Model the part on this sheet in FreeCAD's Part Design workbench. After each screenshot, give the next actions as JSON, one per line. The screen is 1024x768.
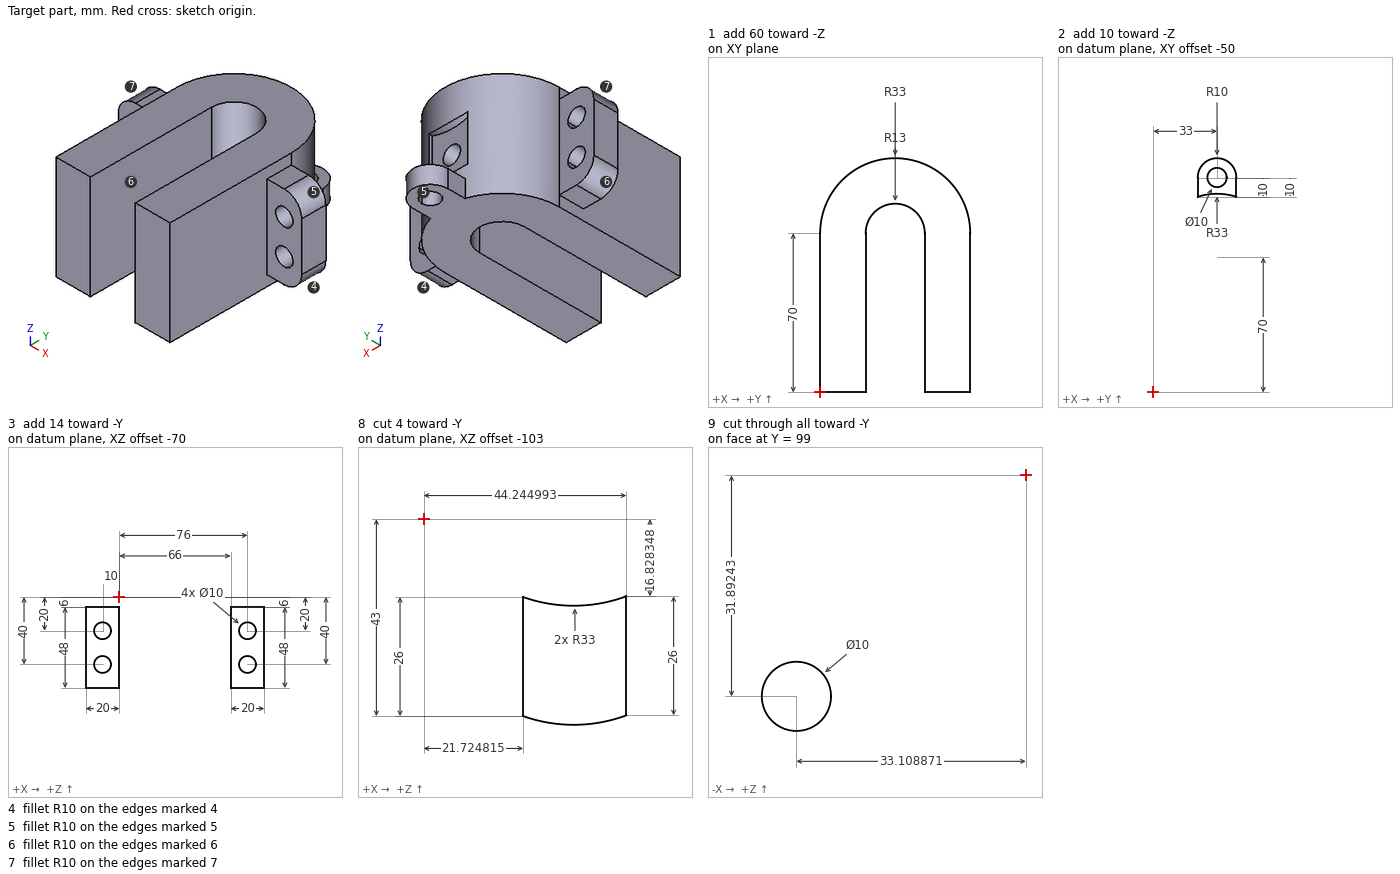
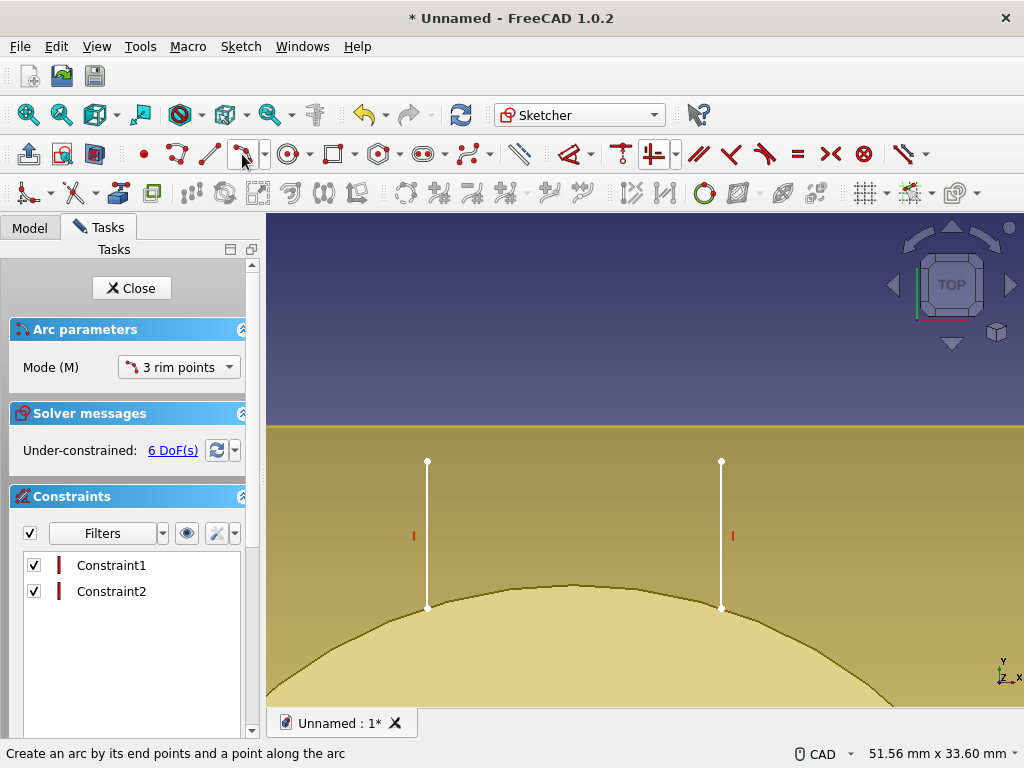
{"action": "left_click", "coordinate": [721, 609]}
{"action": "left_click", "coordinate": [427, 609]}
{"action": "left_click", "coordinate": [574, 585]}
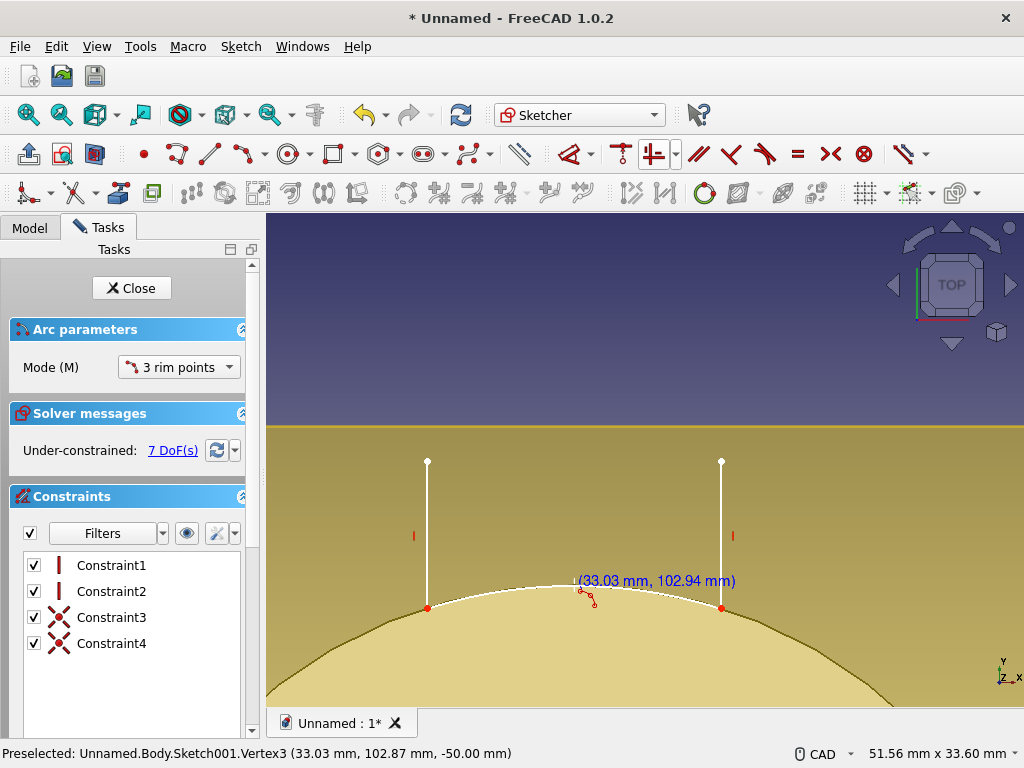
{"action": "left_click", "coordinate": [427, 462]}
{"action": "left_click", "coordinate": [721, 462]}
{"action": "left_click", "coordinate": [574, 314]}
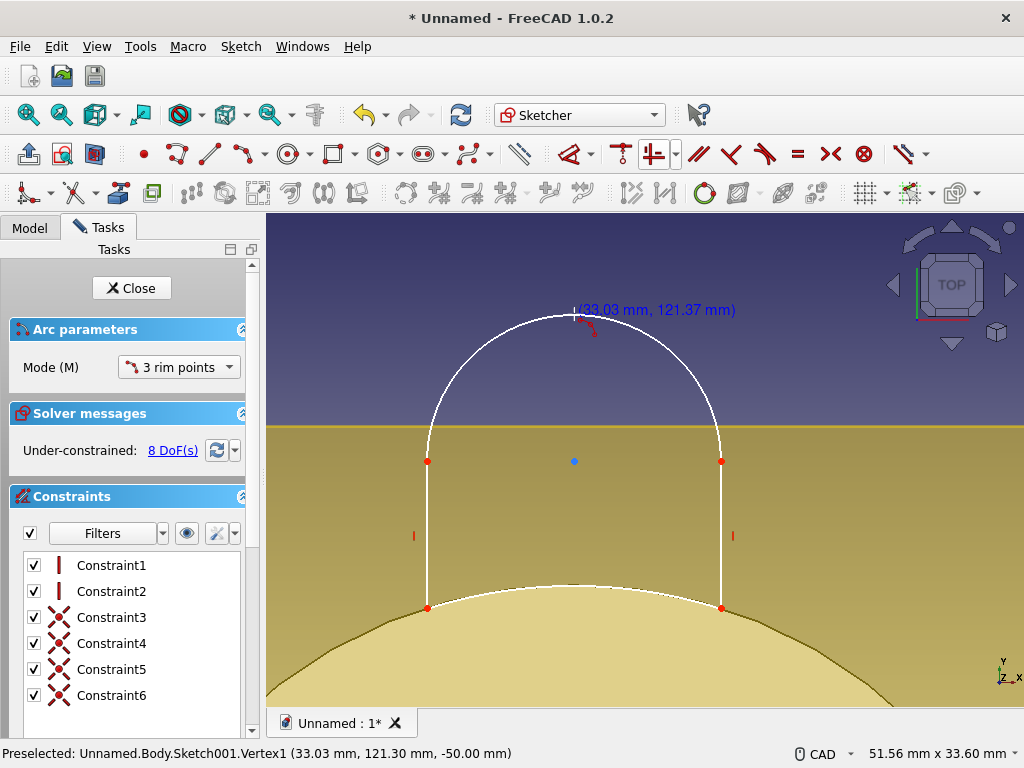
{"action": "key", "text": "g c"}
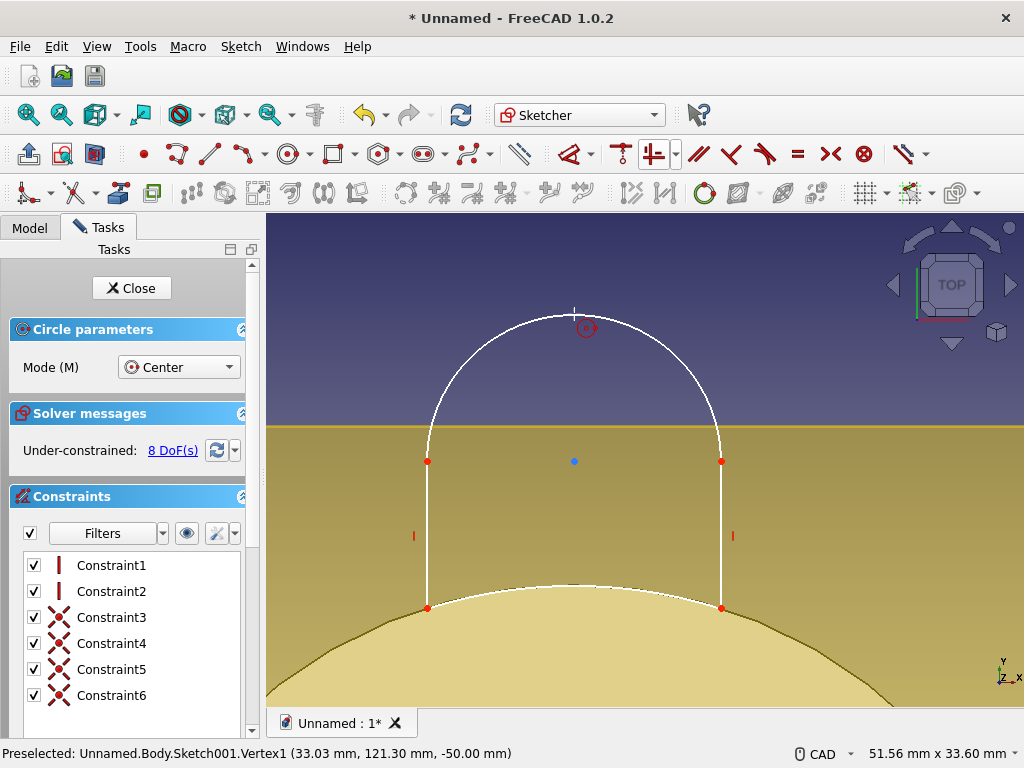
{"action": "left_click", "coordinate": [574, 461]}
{"action": "mouse_move", "coordinate": [626, 409]}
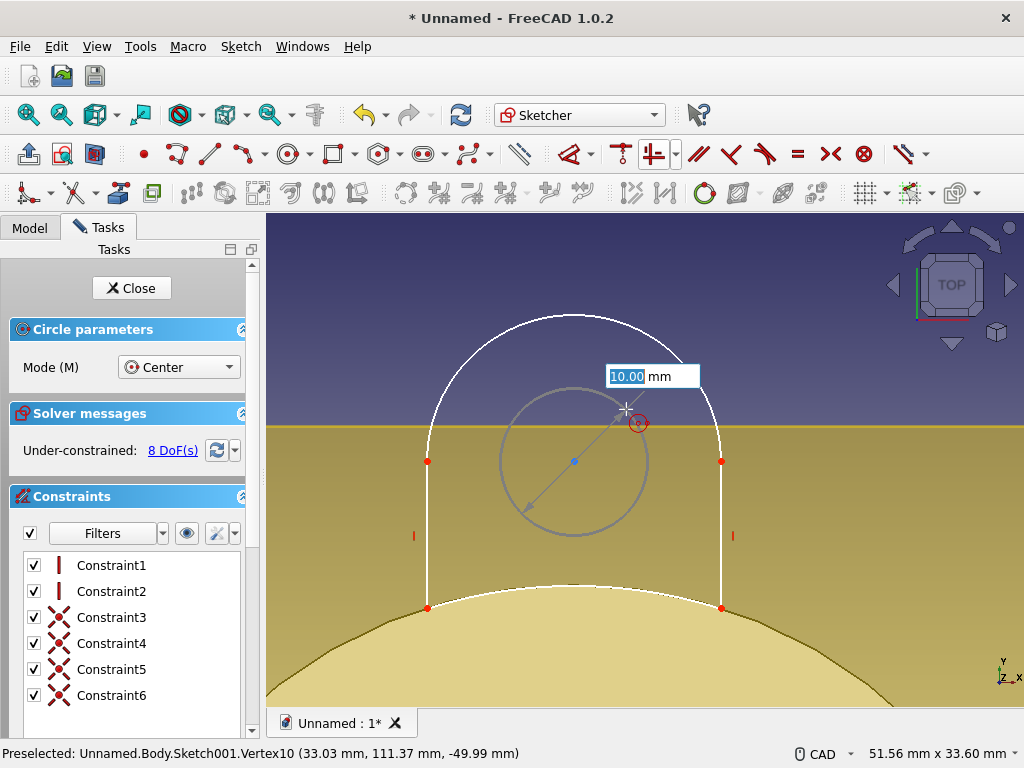
{"action": "type", "text": "10"}
{"action": "key", "text": "Return"}
{"action": "key", "text": "Escape"}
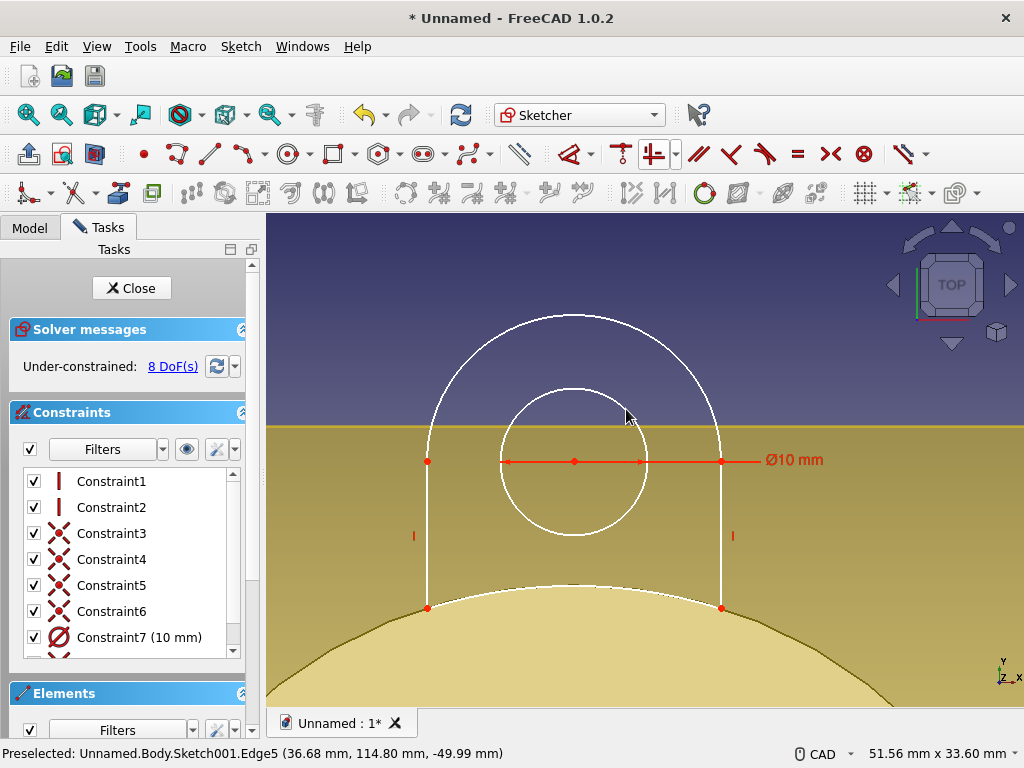
{"action": "left_click", "coordinate": [721, 506]}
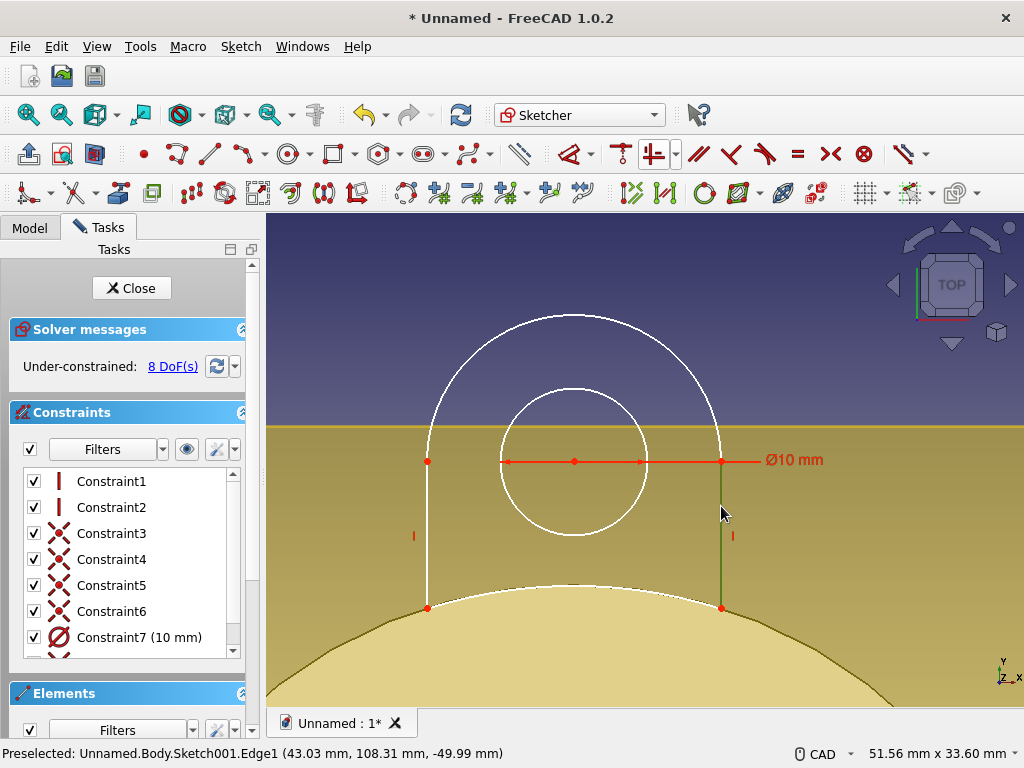
{"action": "left_click", "coordinate": [660, 343]}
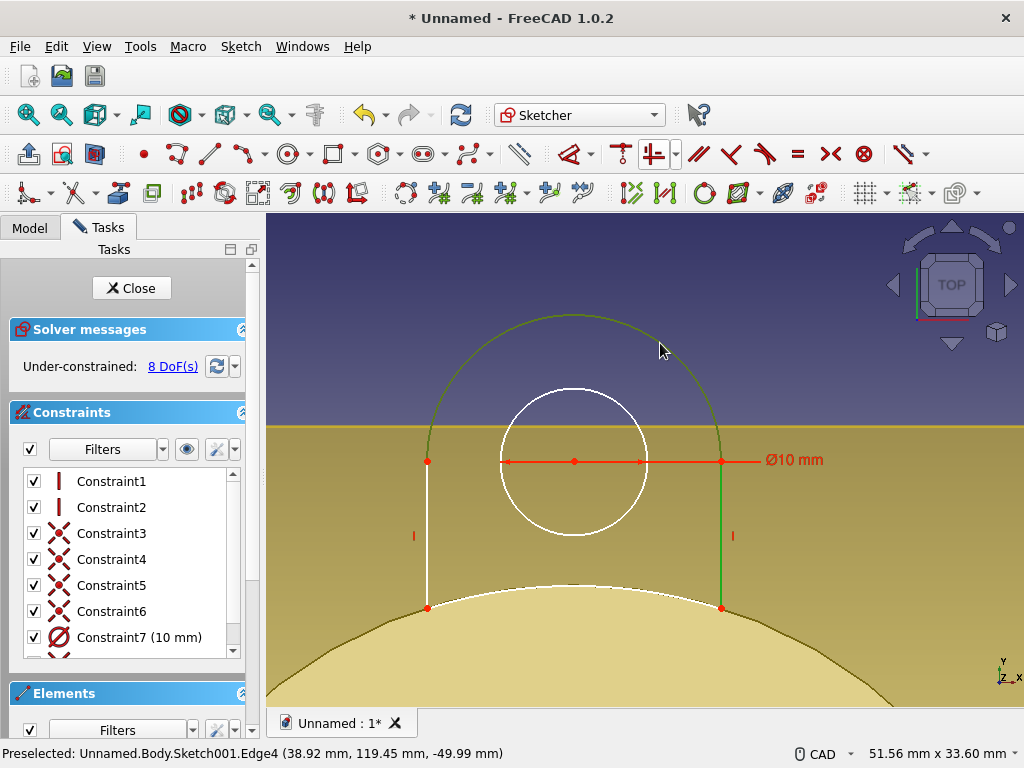
{"action": "left_click", "coordinate": [765, 154]}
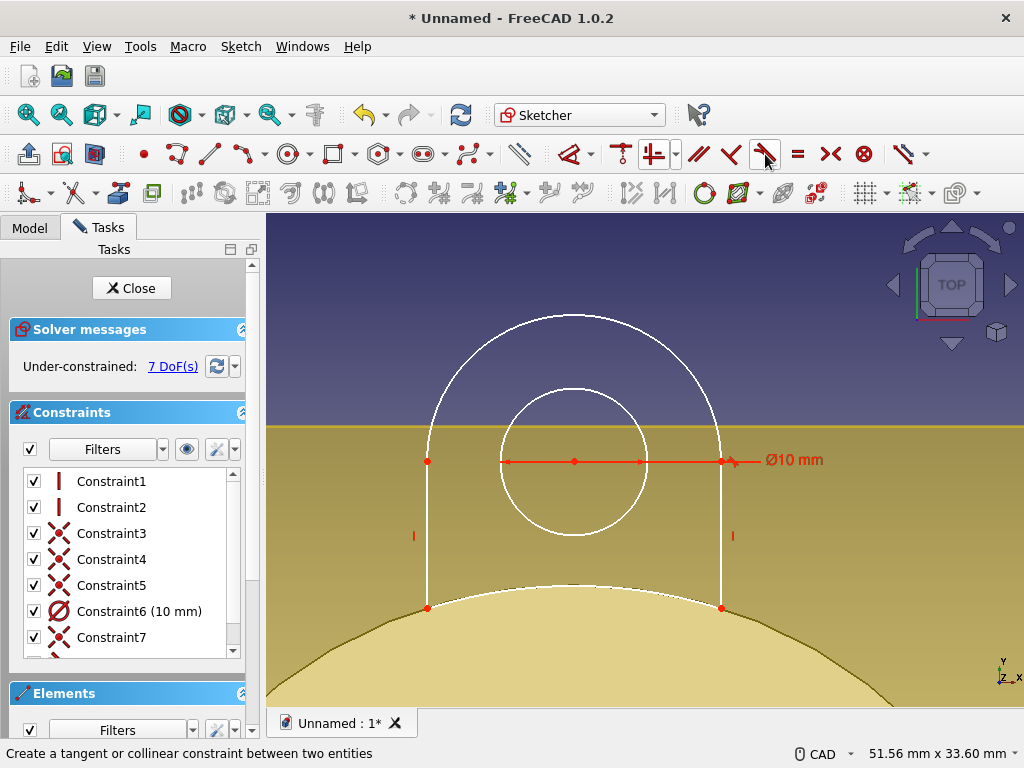
{"action": "left_click", "coordinate": [427, 565]}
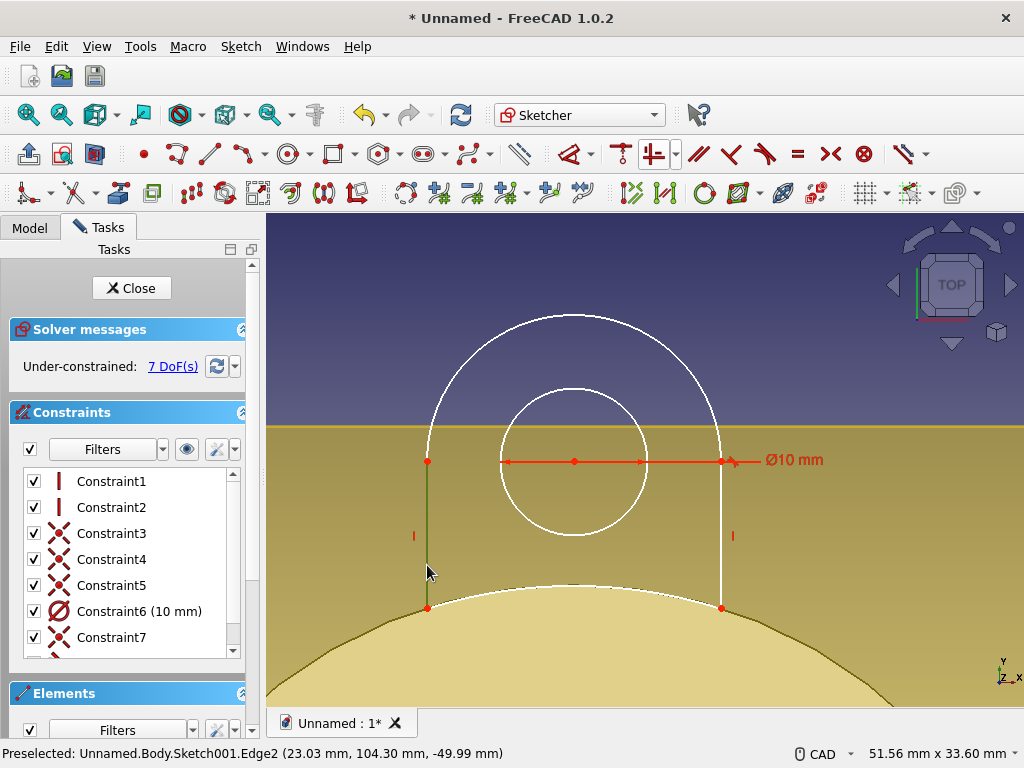
{"action": "left_click", "coordinate": [660, 343]}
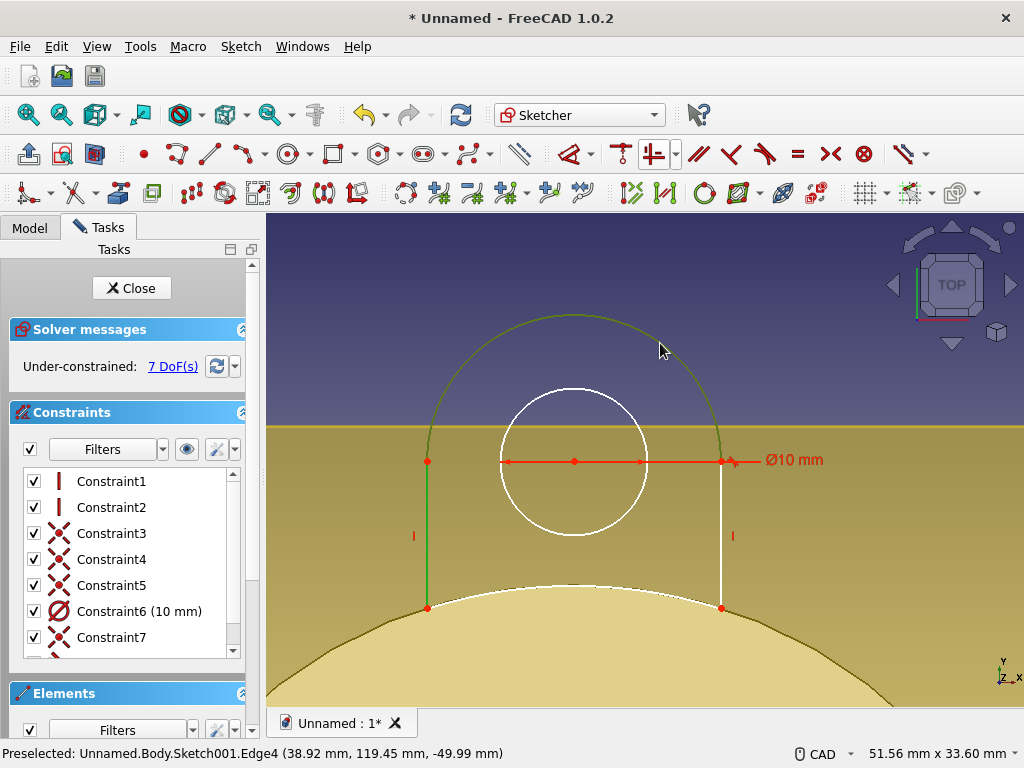
{"action": "left_click", "coordinate": [765, 154]}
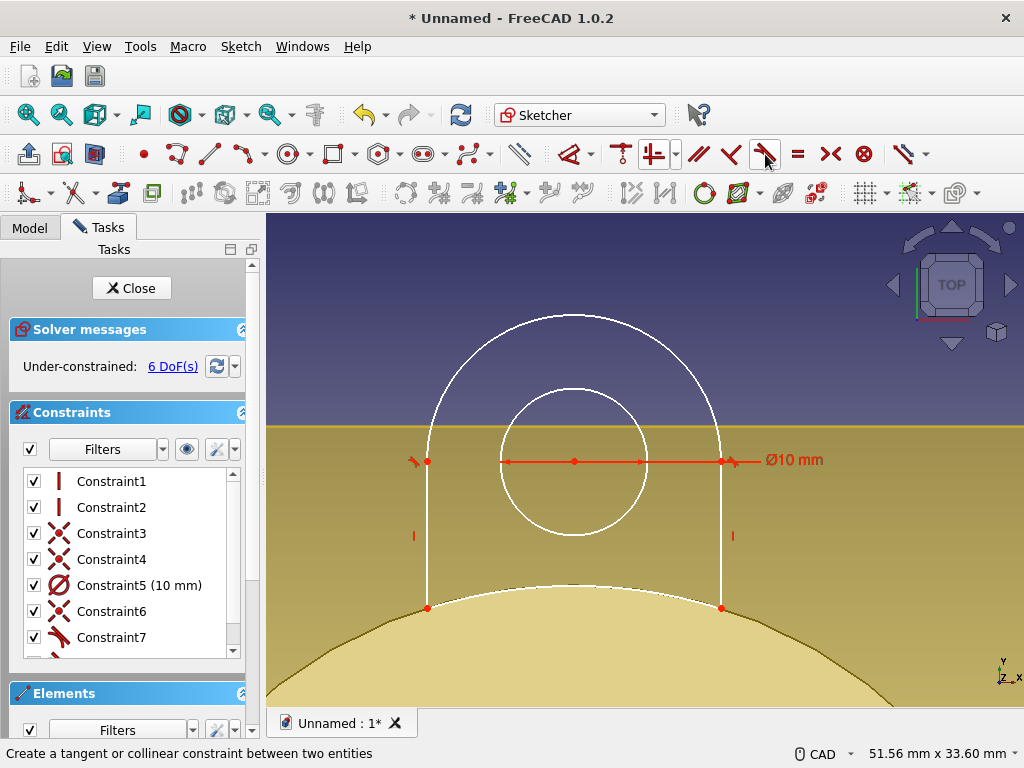
{"action": "key", "text": "d"}